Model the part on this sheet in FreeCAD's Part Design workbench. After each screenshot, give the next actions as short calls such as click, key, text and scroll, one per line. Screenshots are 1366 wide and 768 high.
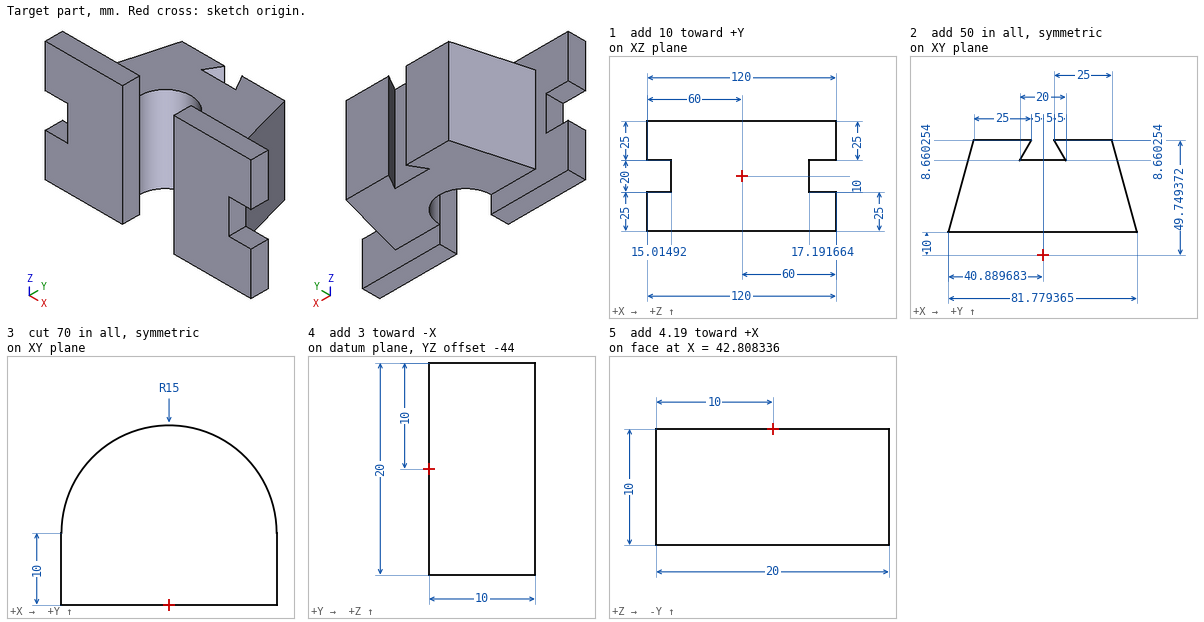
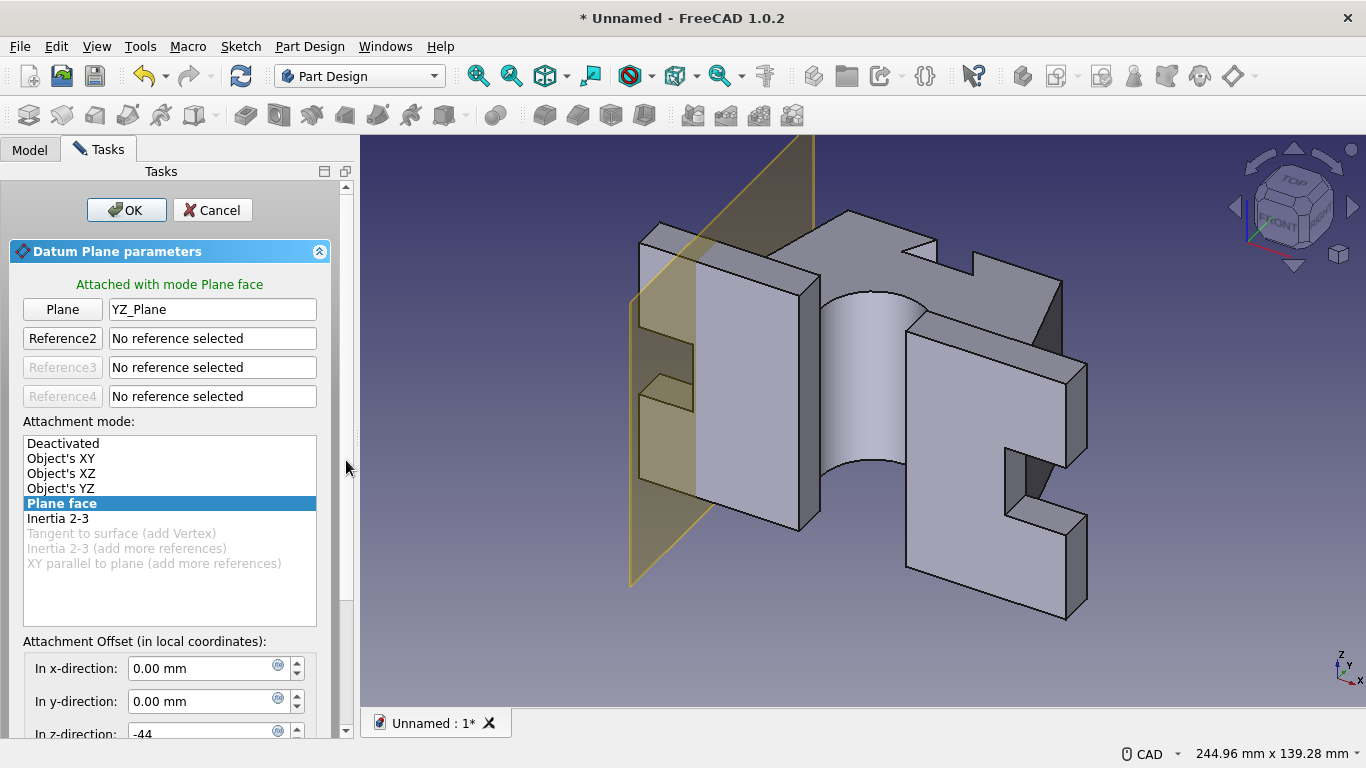
click(127, 210)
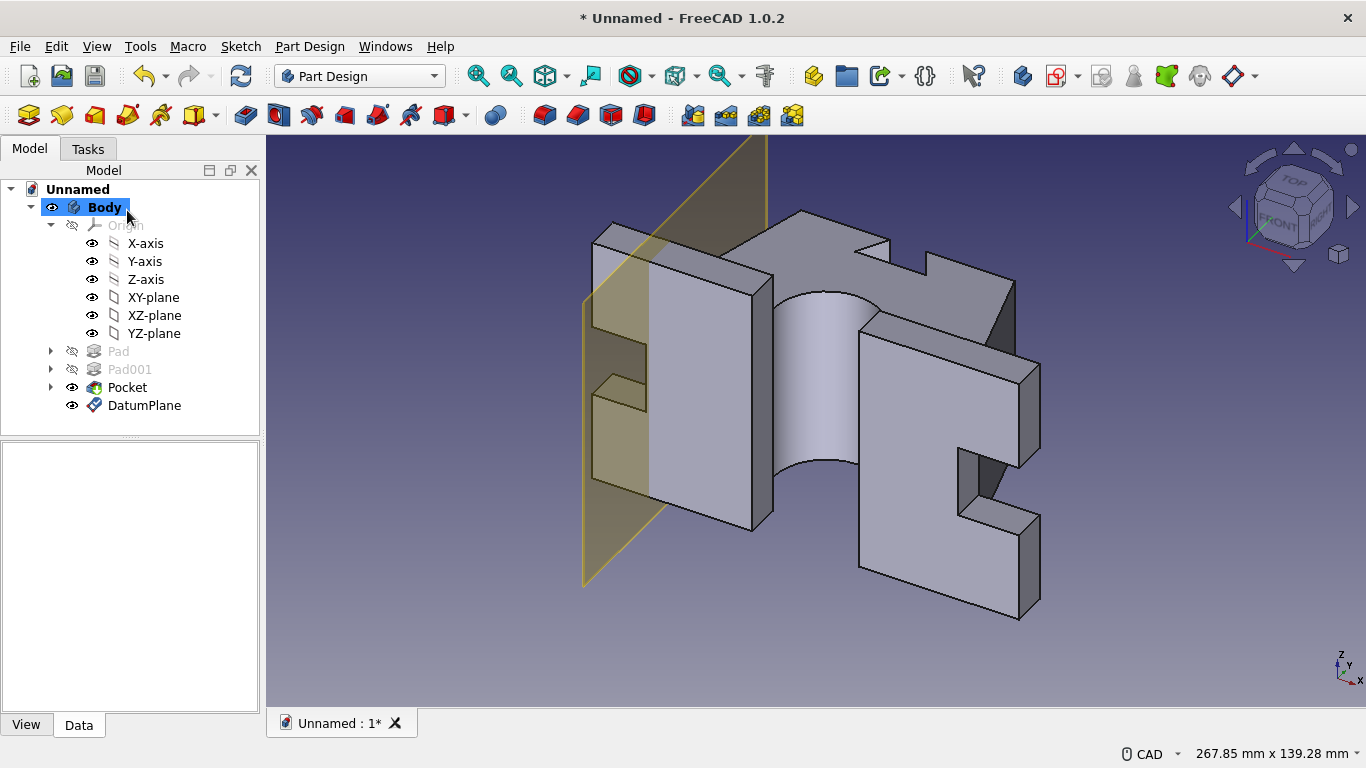
click(117, 405)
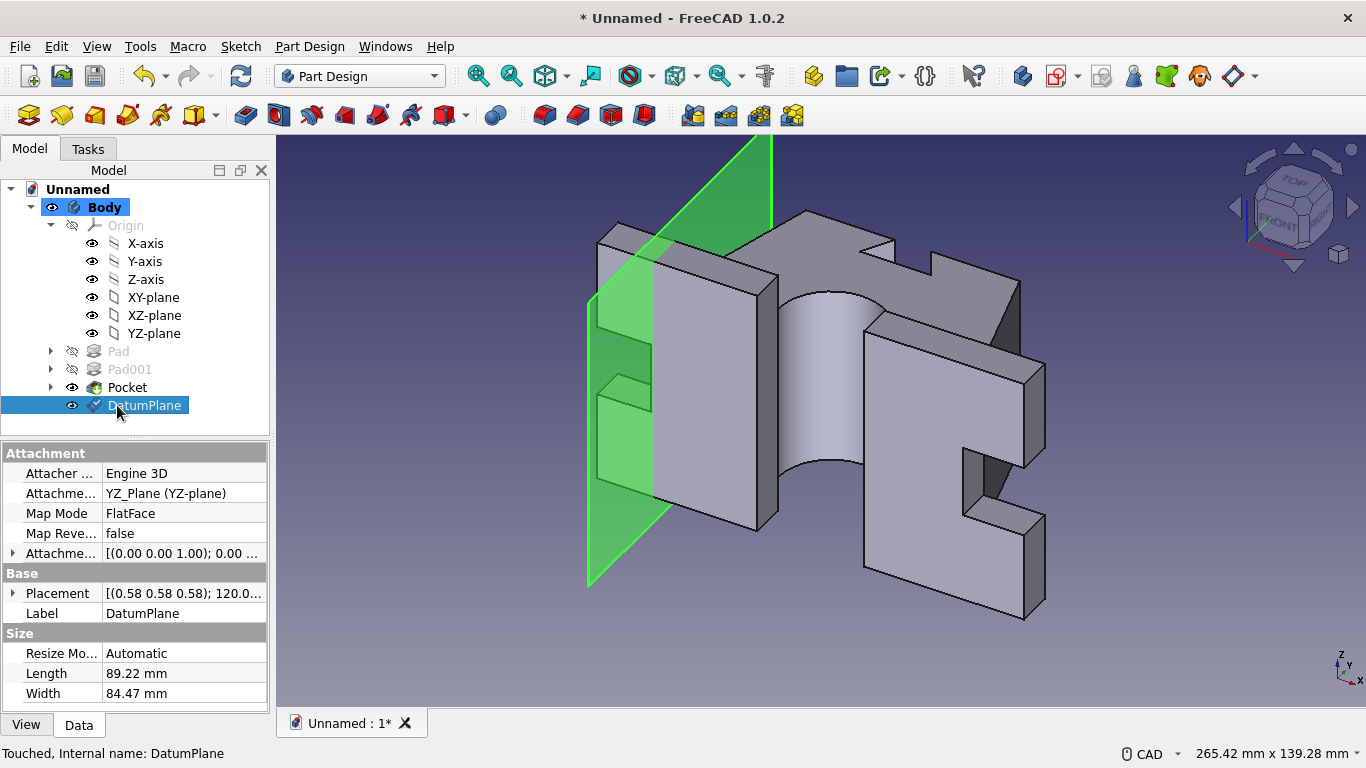
click(1056, 76)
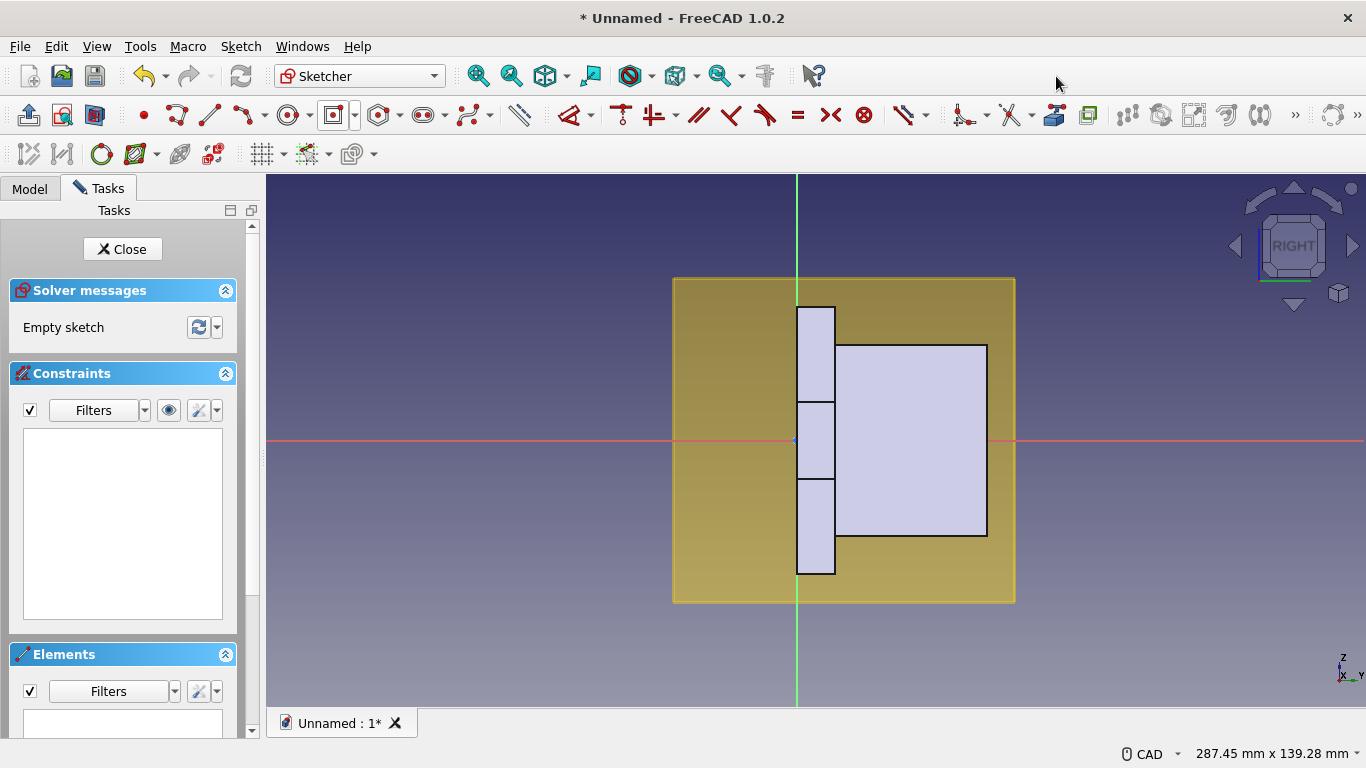
key(q)
key(s)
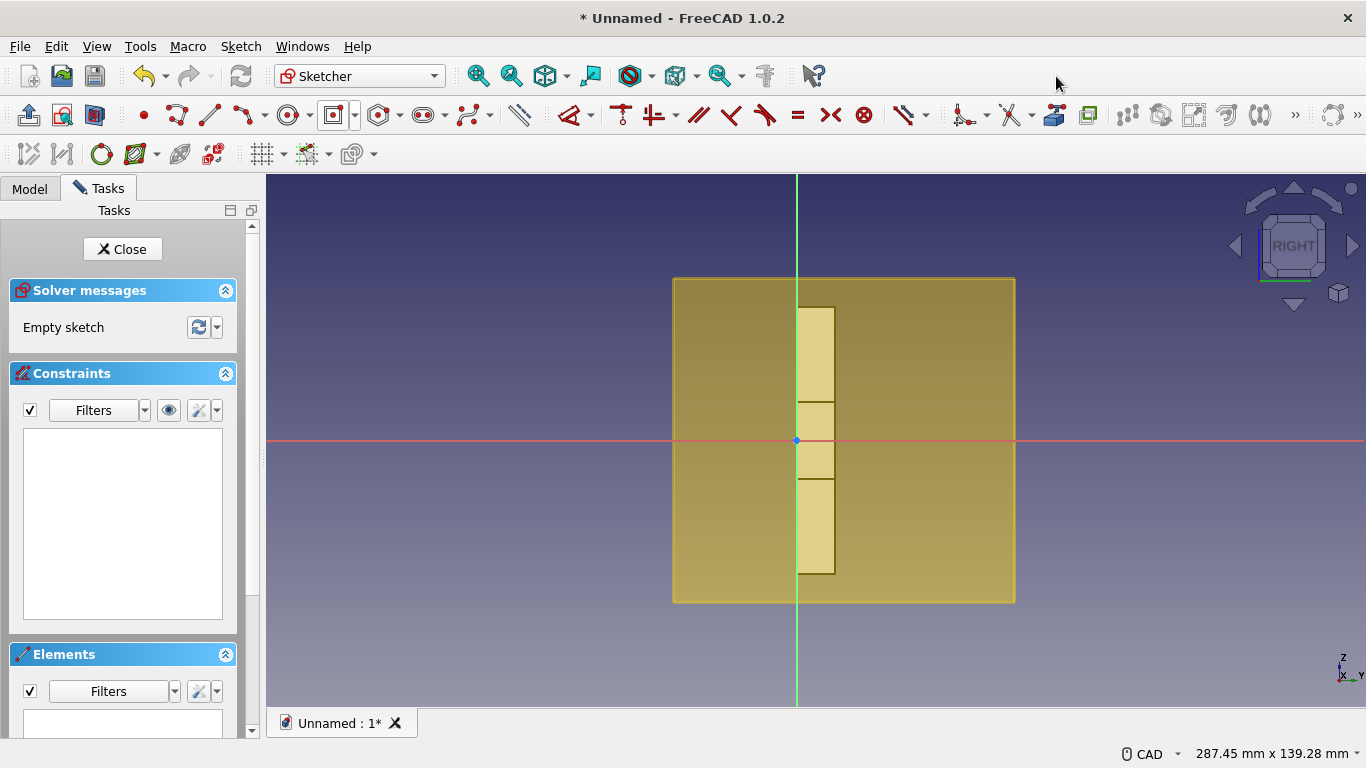
scroll(838, 440, up, 7)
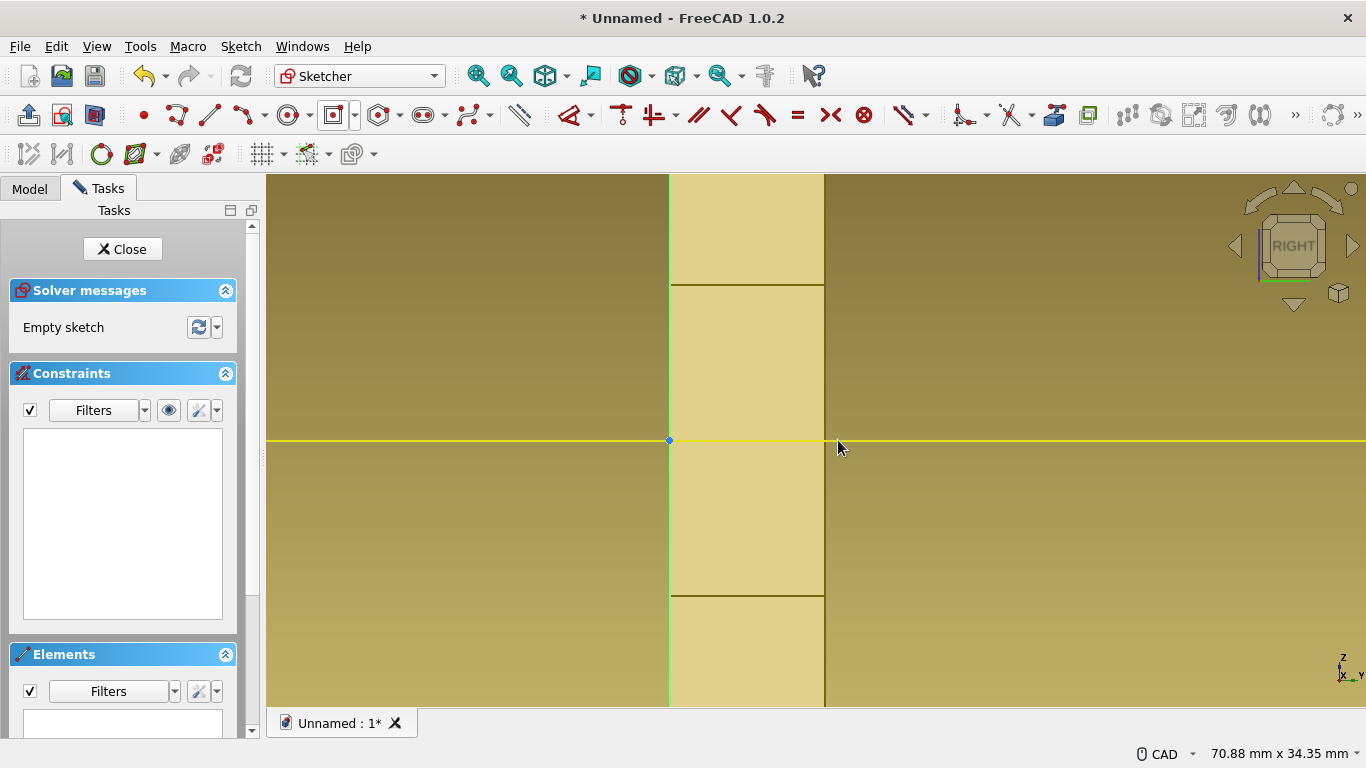
key(g)
key(r)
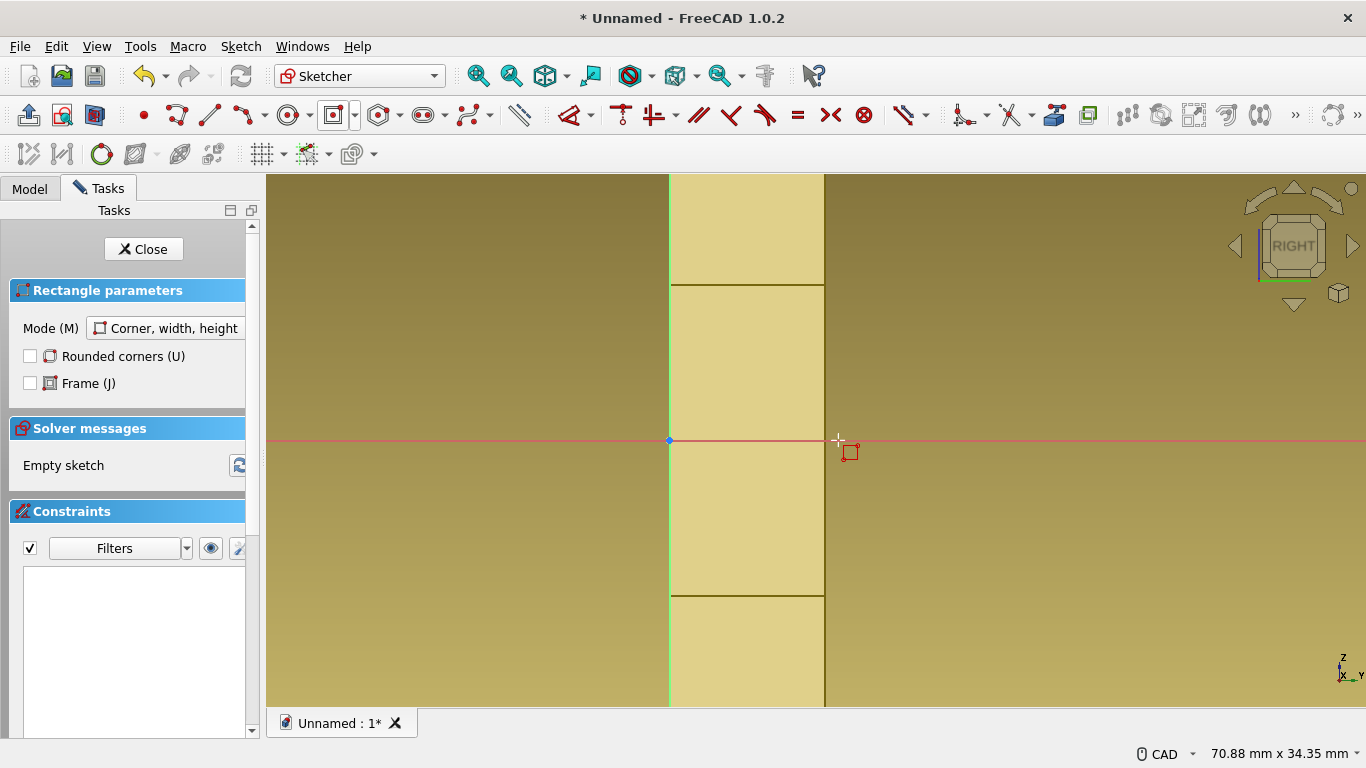
click(670, 285)
click(825, 596)
key(Escape)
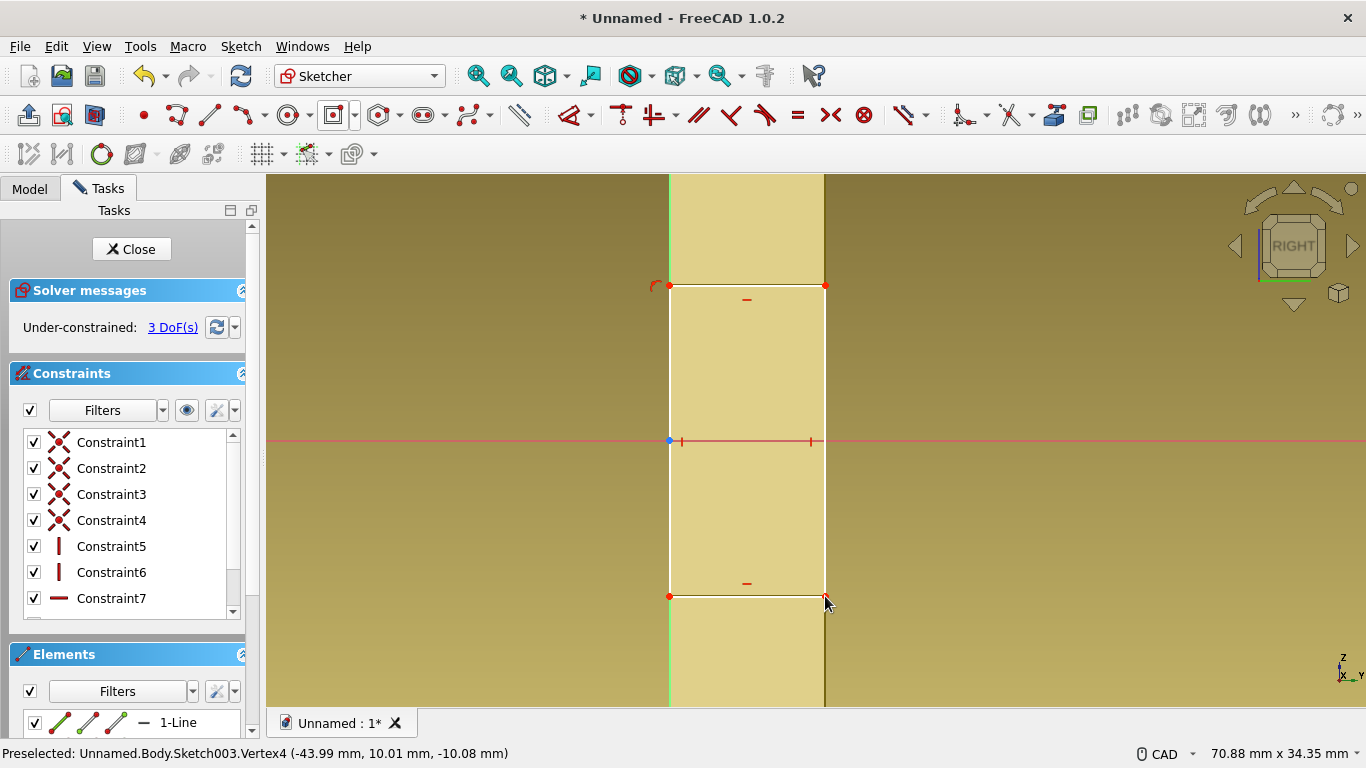
key(d)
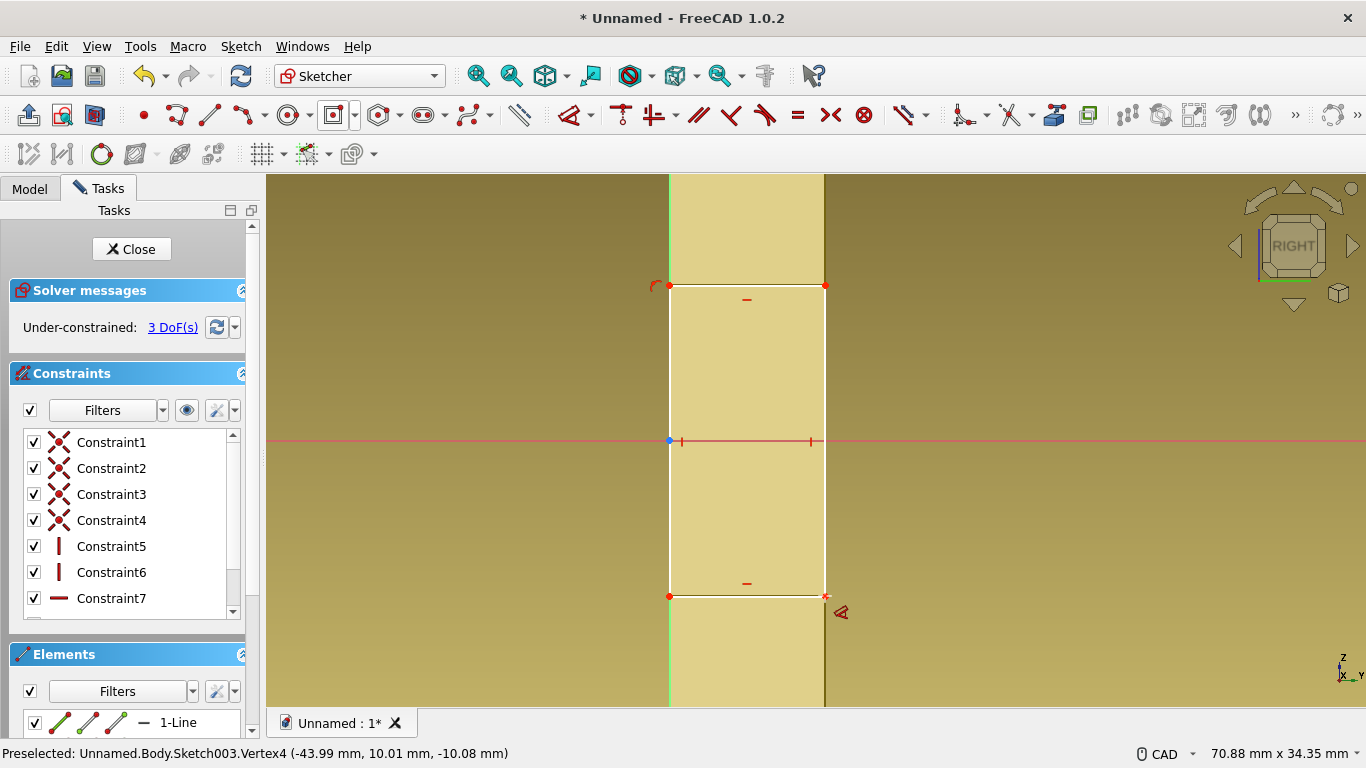
click(670, 379)
click(636, 370)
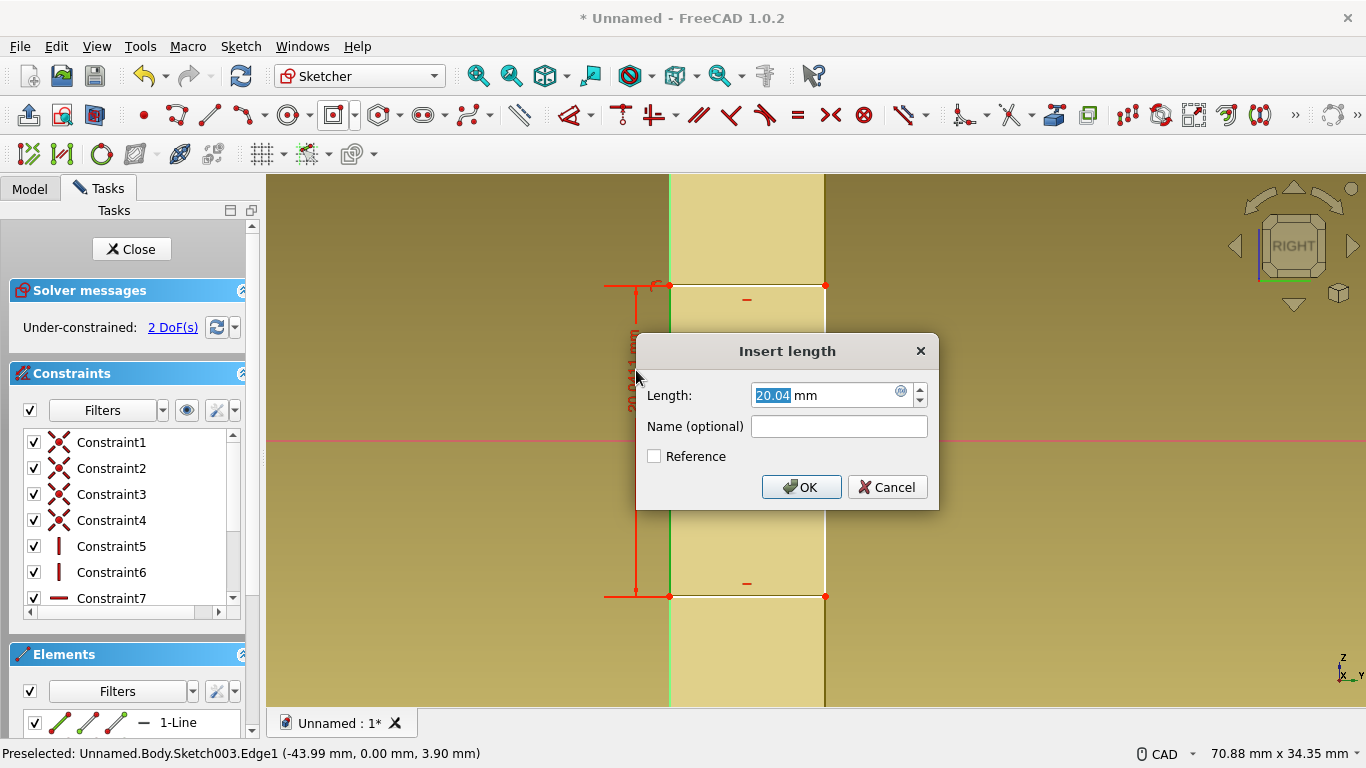
text(20)
key(Return)